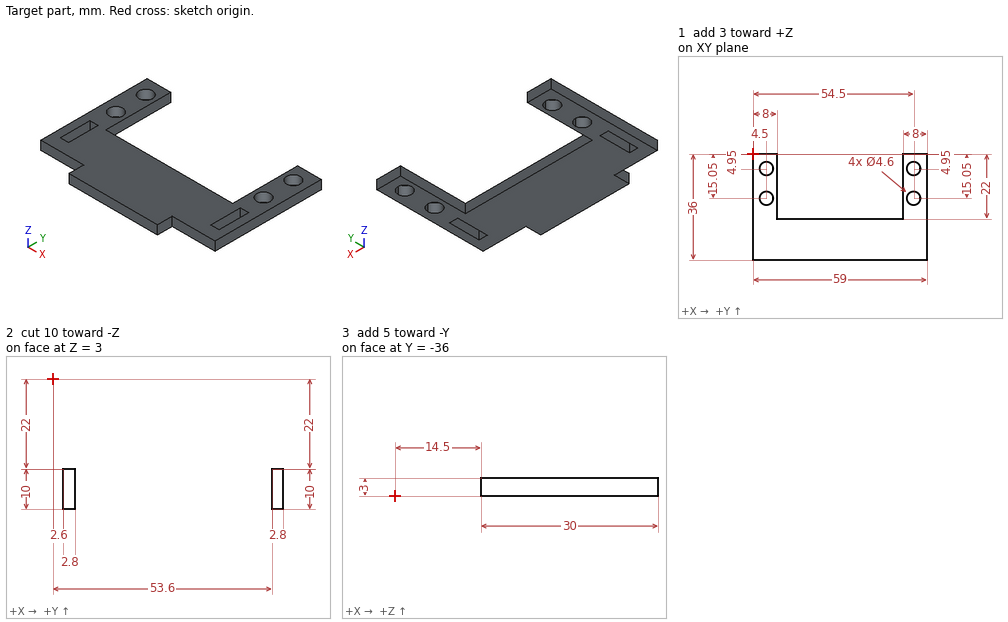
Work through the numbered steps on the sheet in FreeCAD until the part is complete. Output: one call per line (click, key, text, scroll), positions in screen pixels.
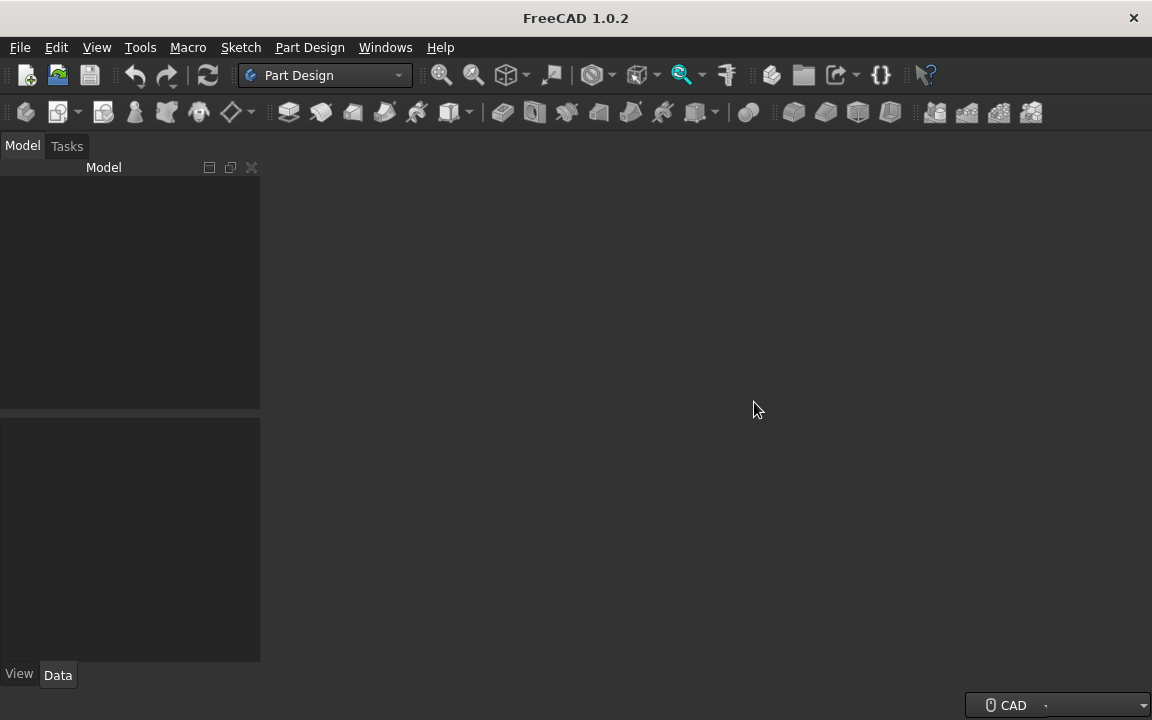
click(26, 76)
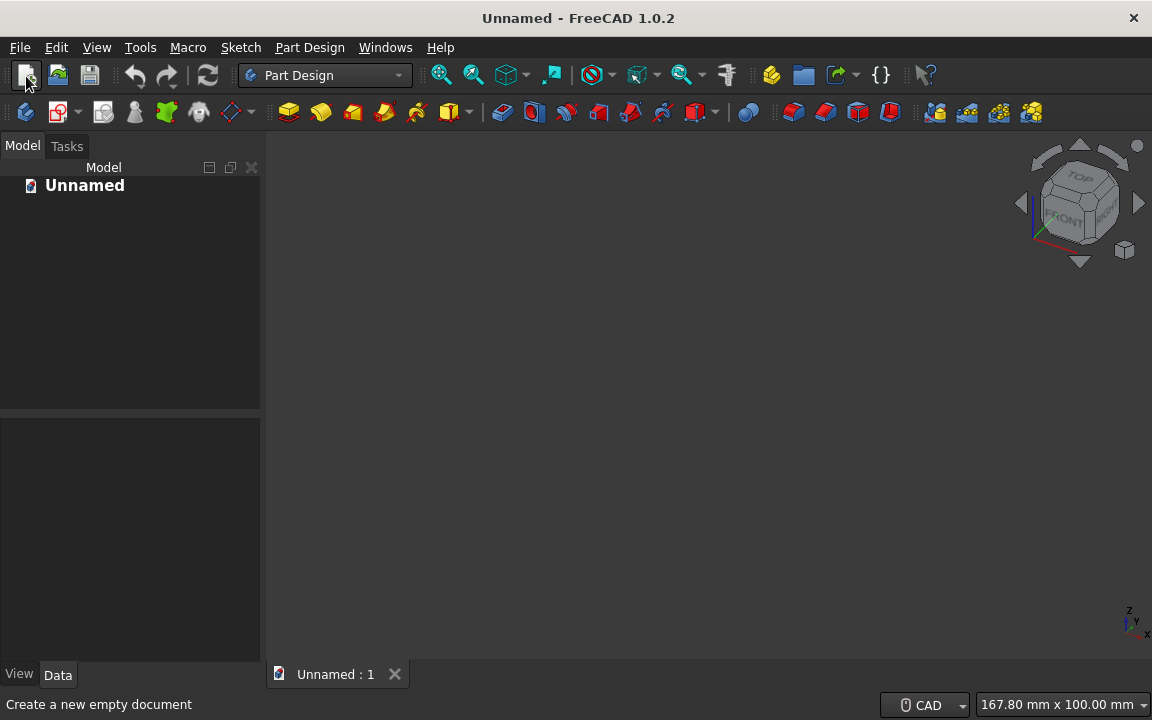
click(58, 112)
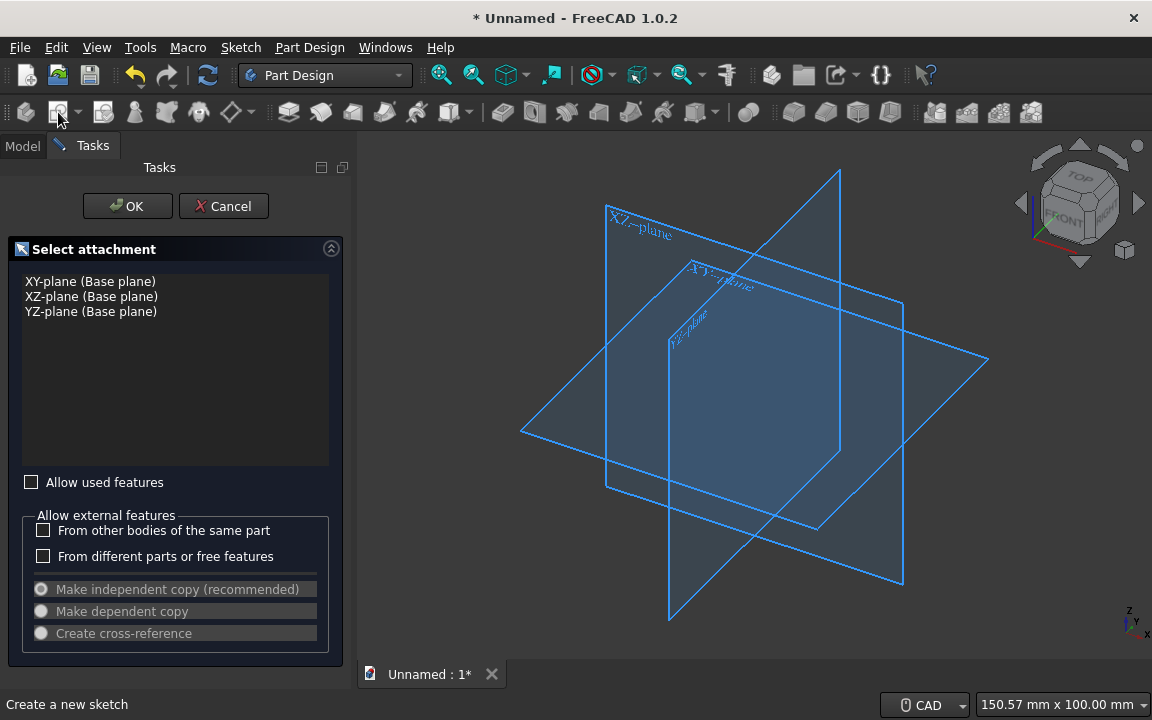
click(82, 282)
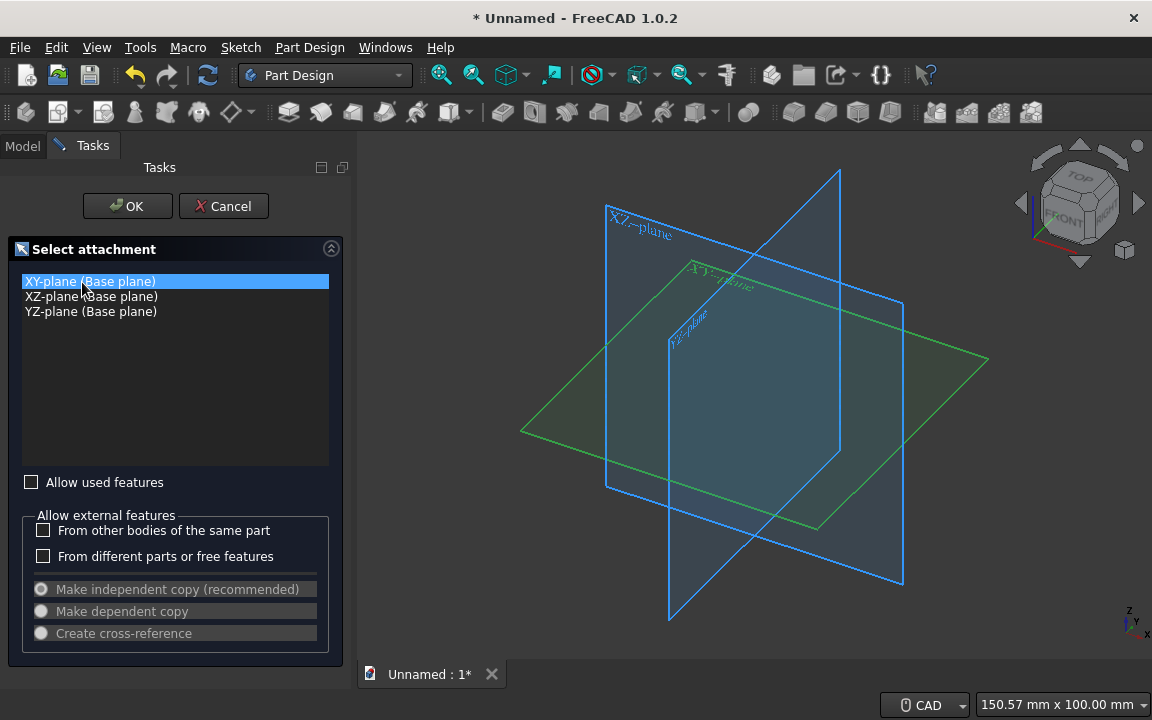
click(128, 206)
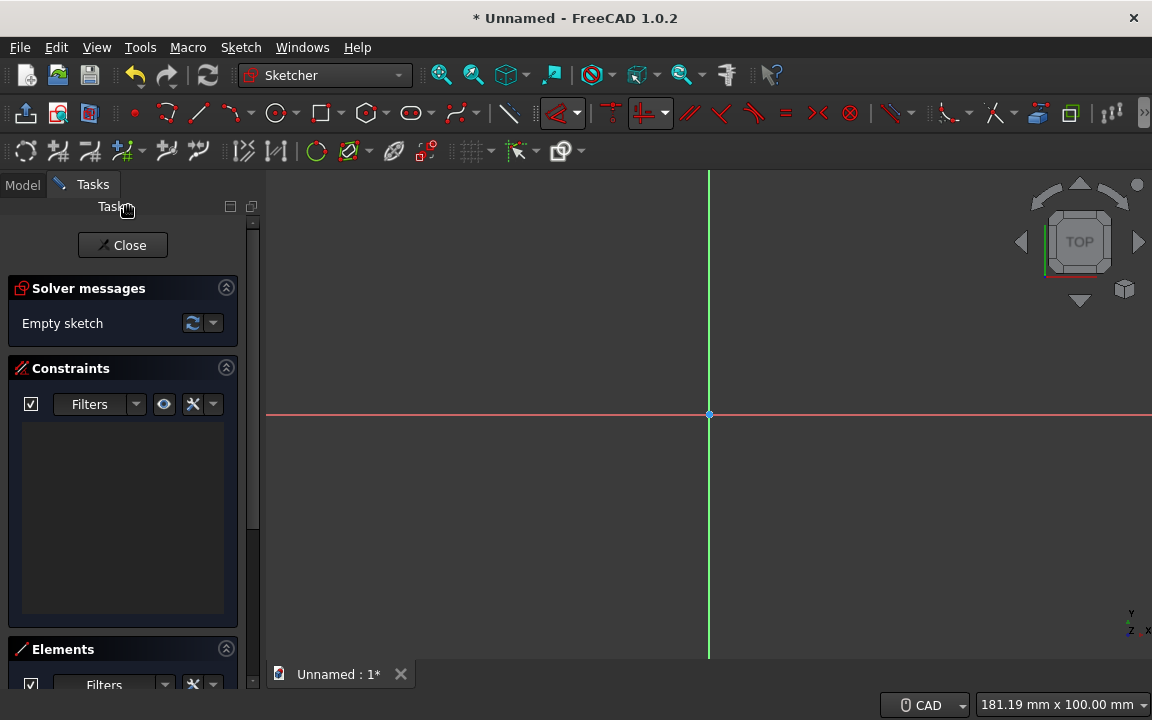
scroll(640, 414, down, 5)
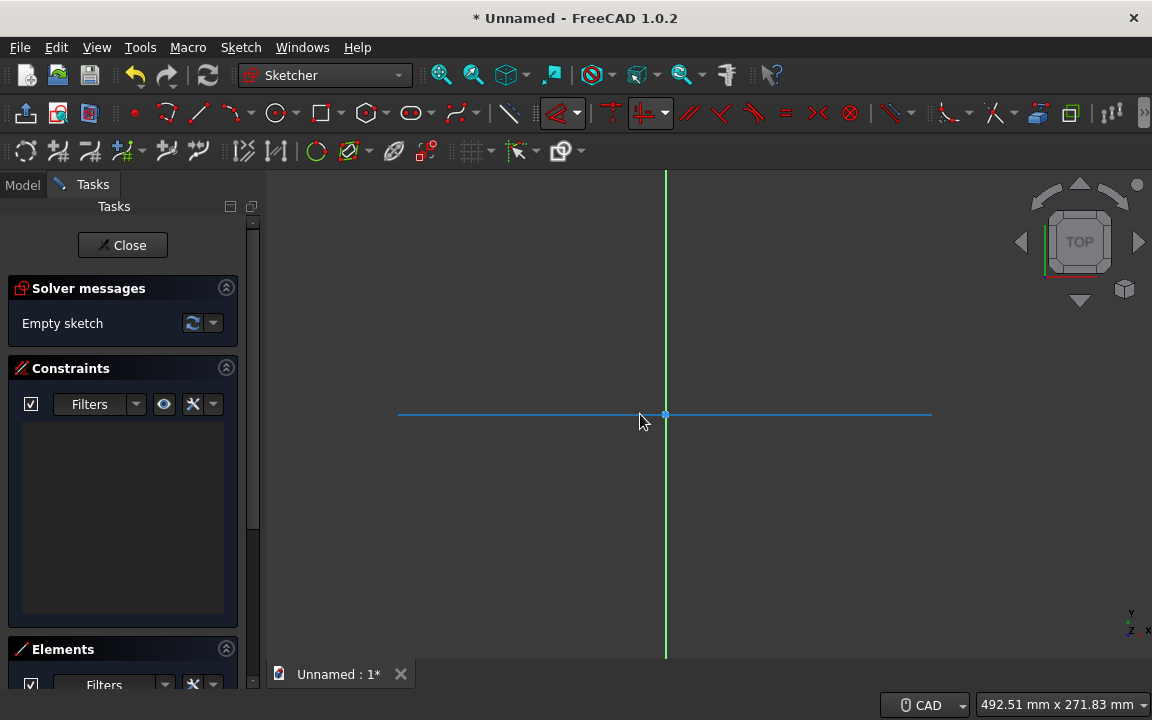
scroll(739, 455, up, 8)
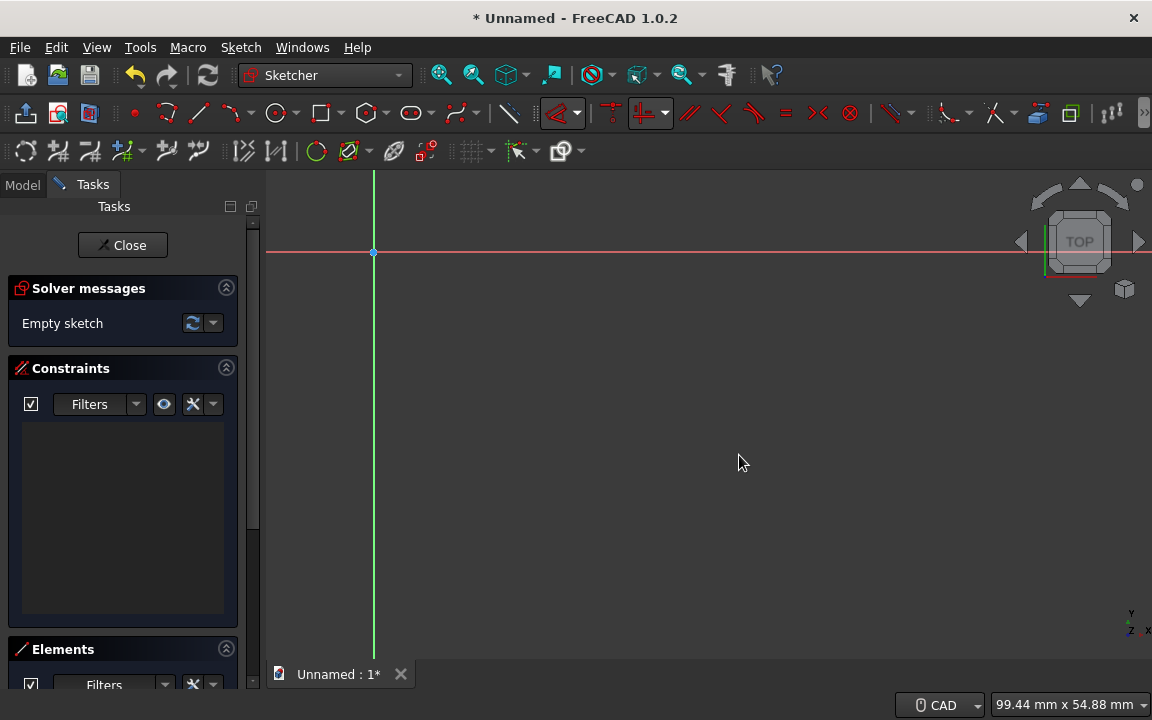
key(g)
key(m)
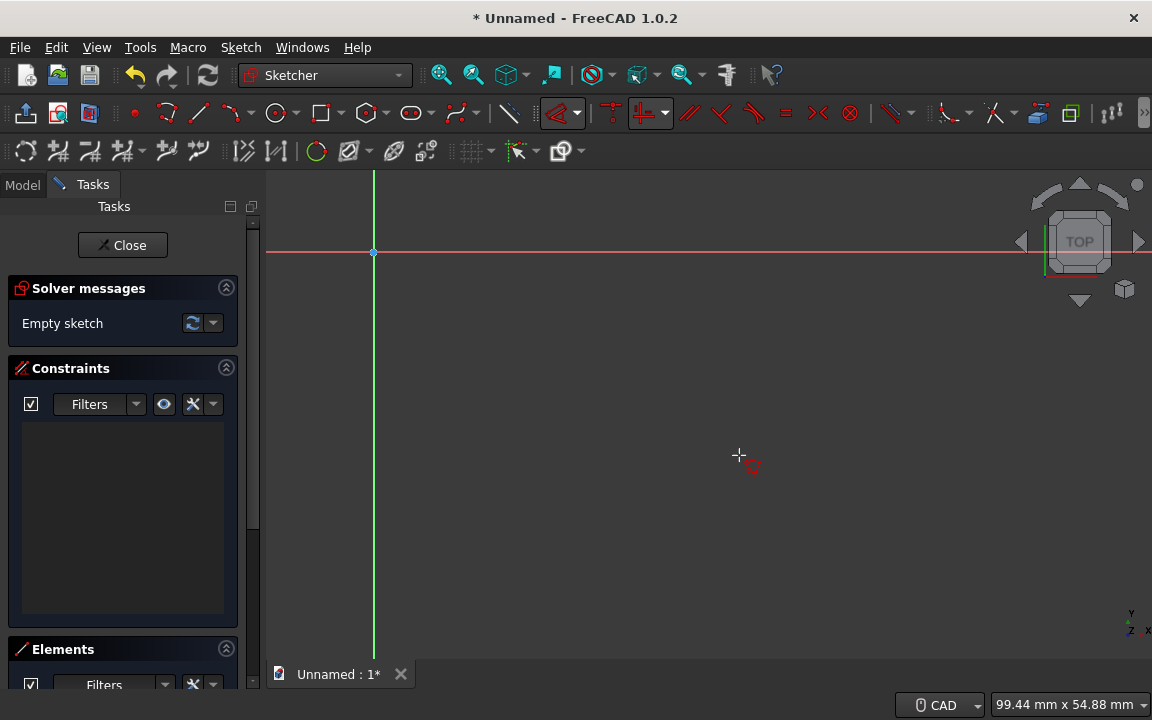
click(374, 252)
click(383, 573)
click(899, 573)
click(899, 252)
click(828, 261)
click(828, 448)
click(445, 448)
click(445, 261)
click(374, 252)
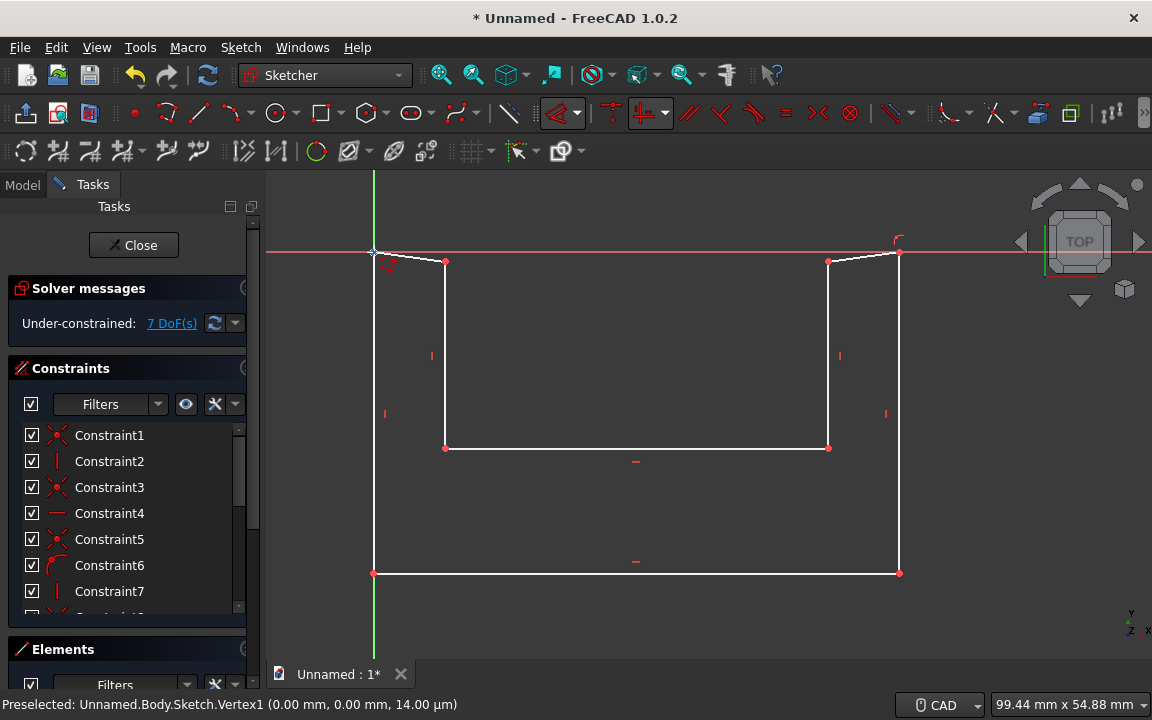
click(276, 114)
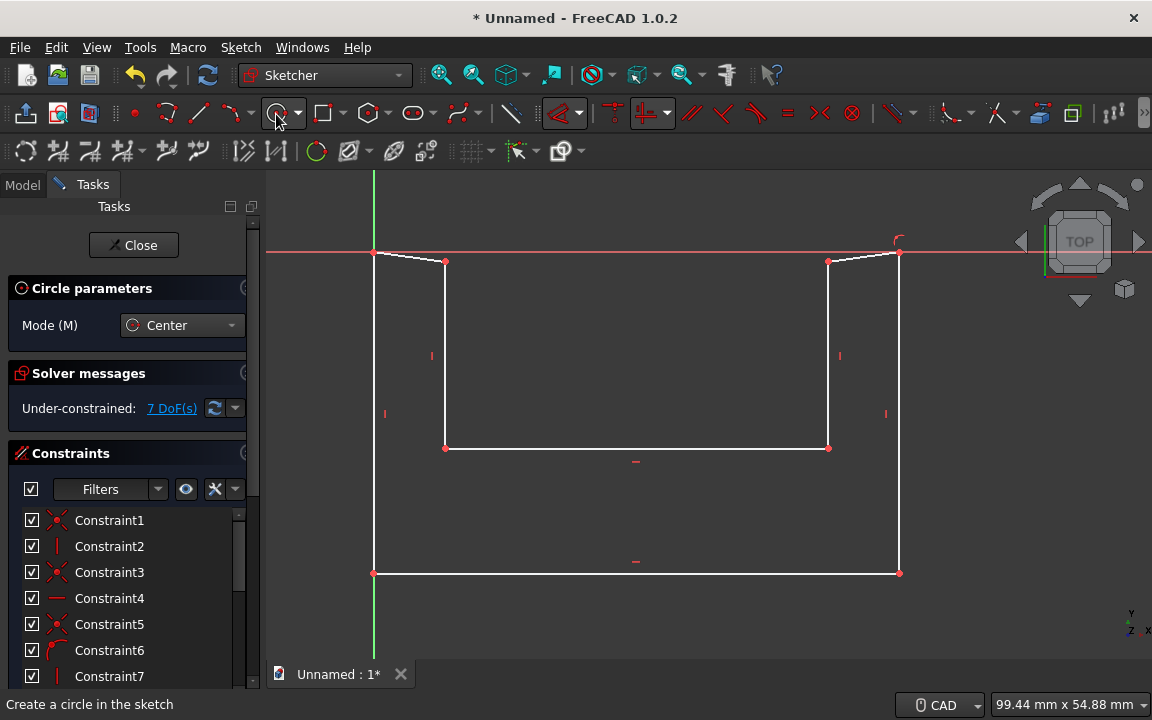
click(859, 386)
click(874, 372)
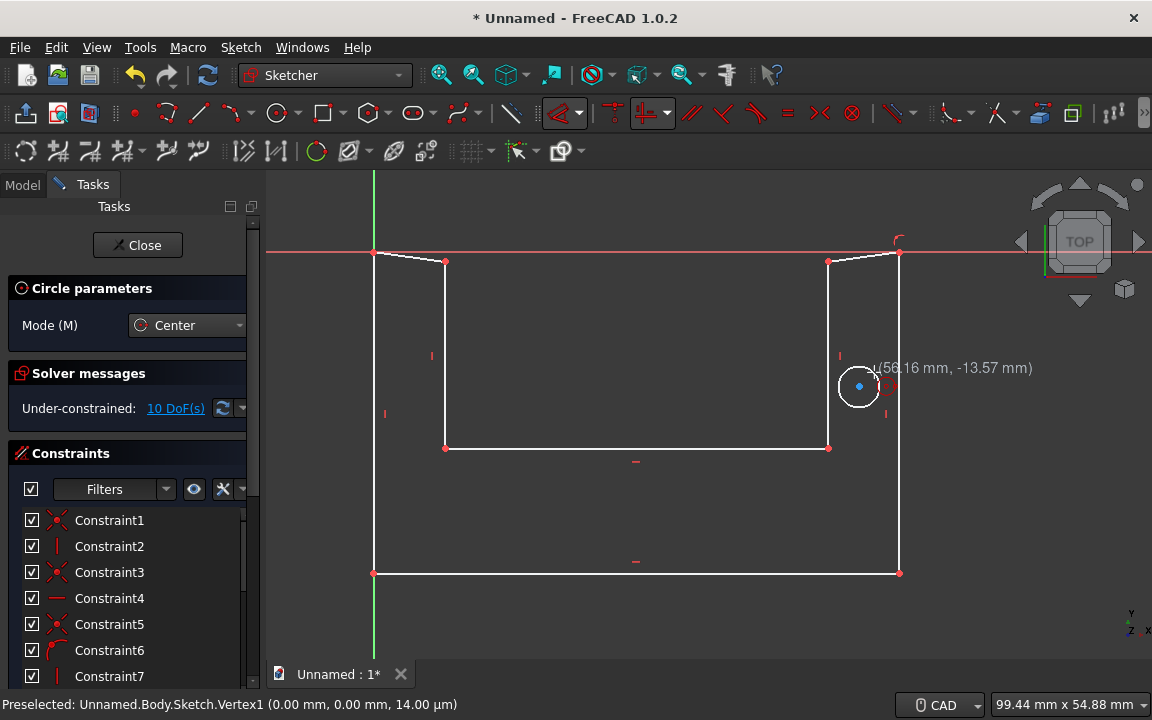
click(414, 386)
click(428, 372)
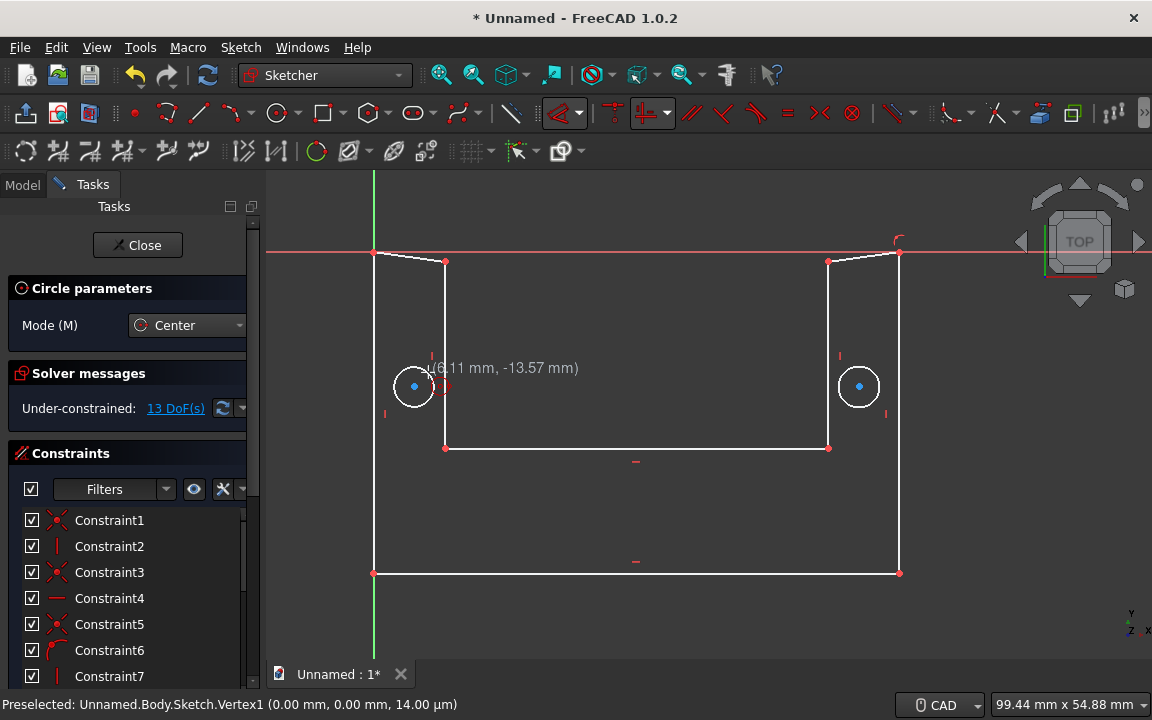
click(859, 296)
click(874, 282)